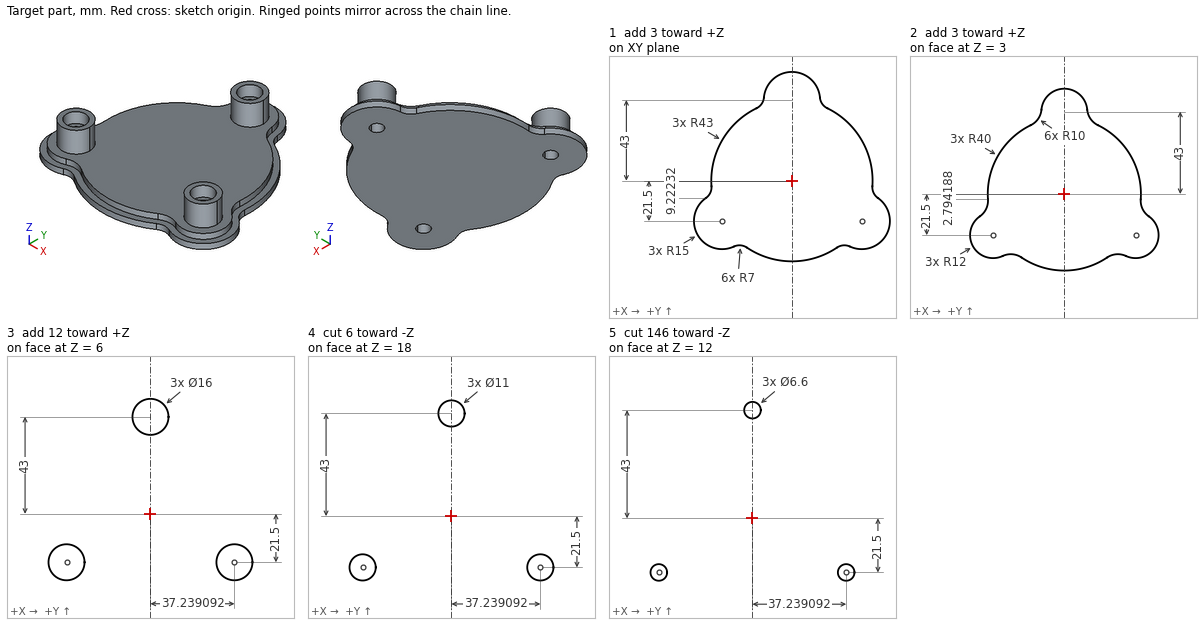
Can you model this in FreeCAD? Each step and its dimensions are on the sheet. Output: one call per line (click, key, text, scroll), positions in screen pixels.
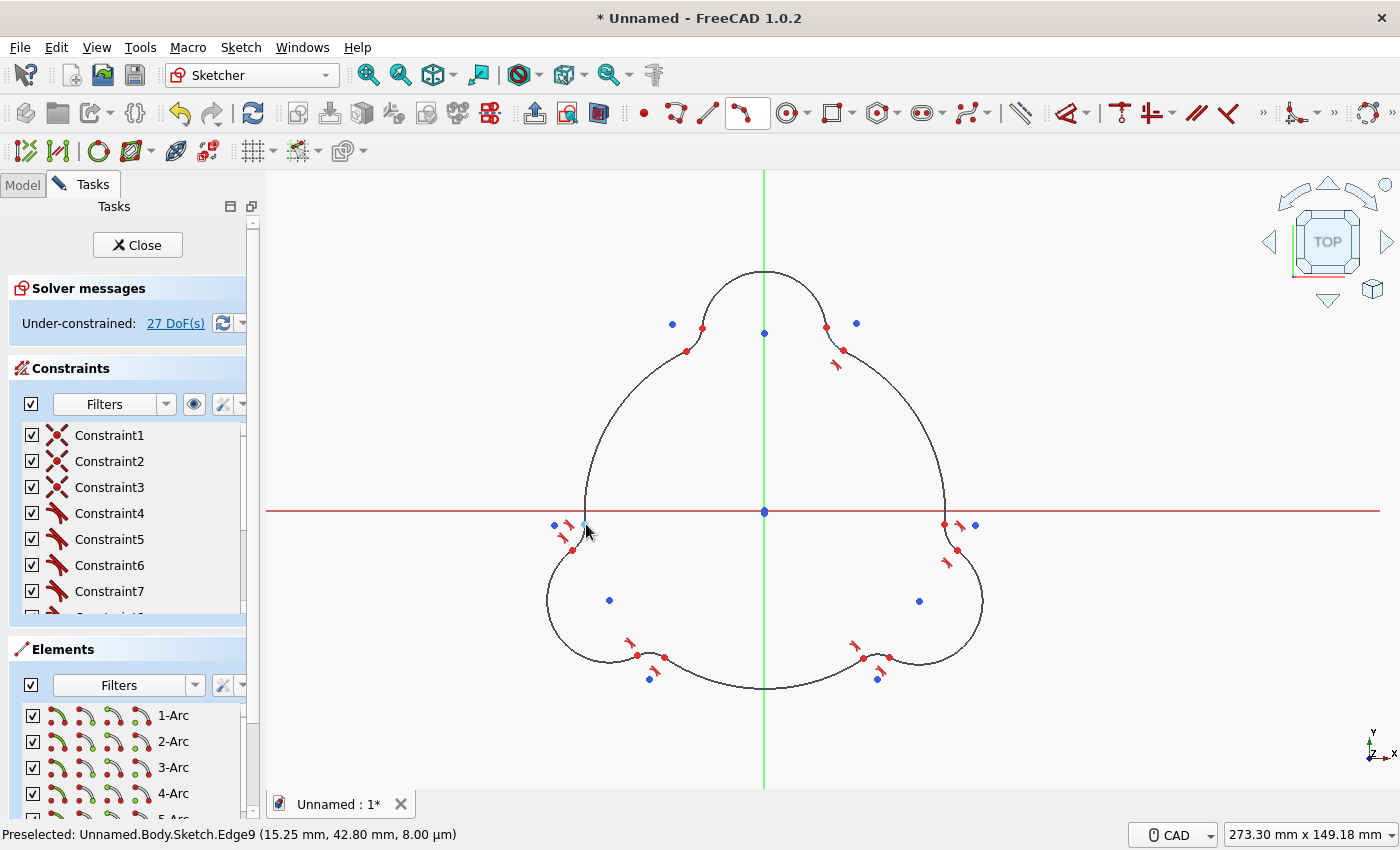
click(799, 282)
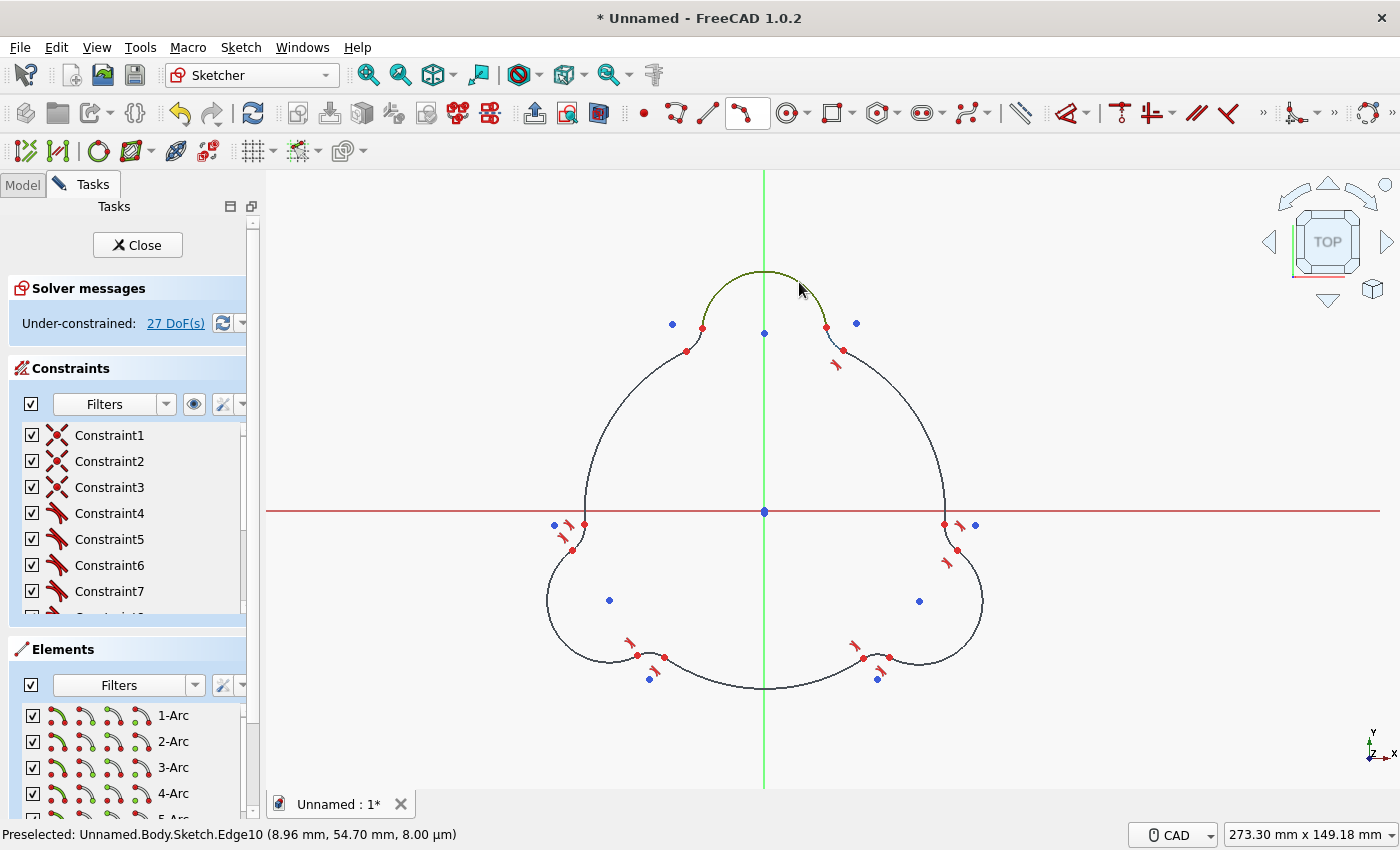
key(t)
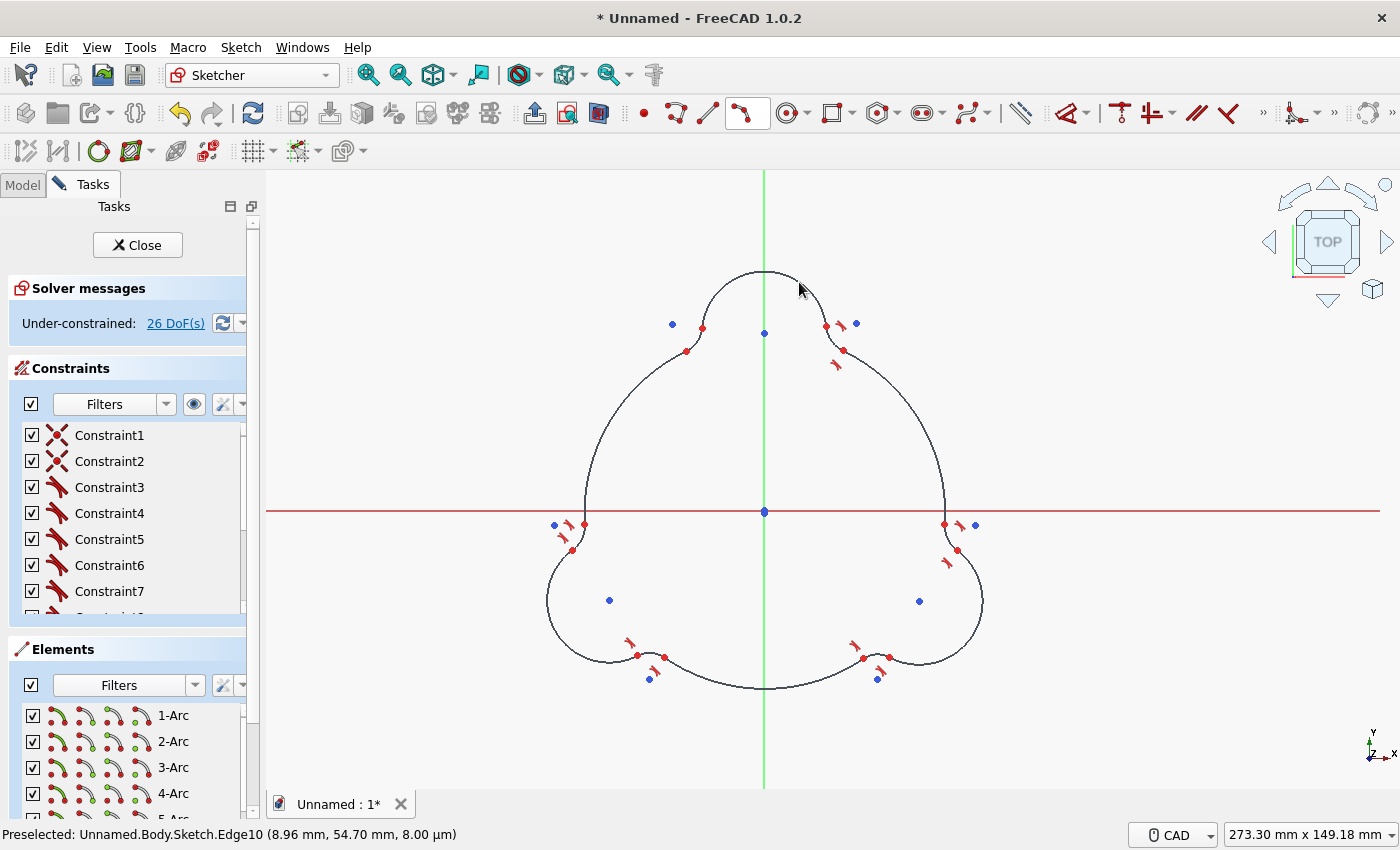
click(798, 282)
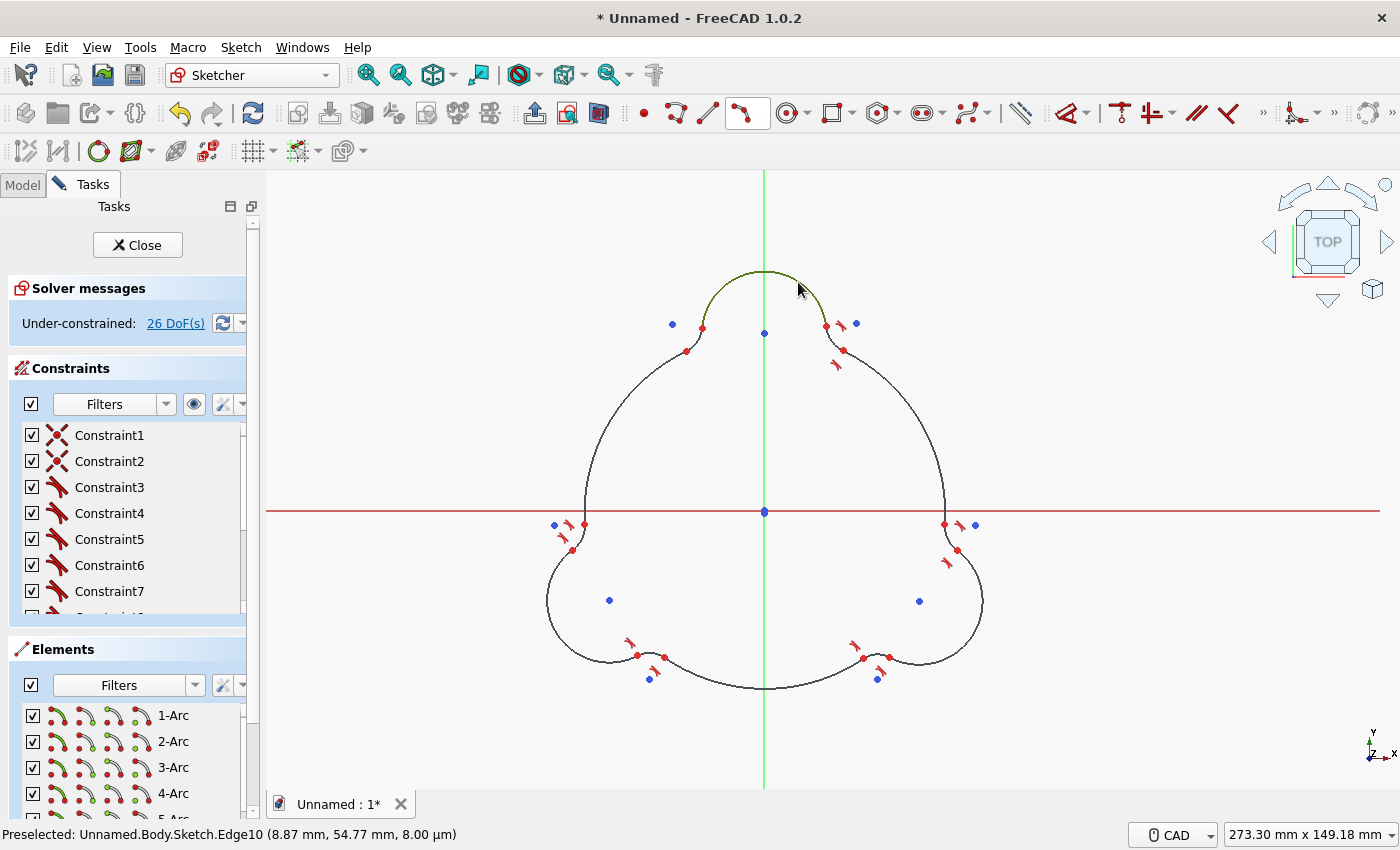
click(697, 342)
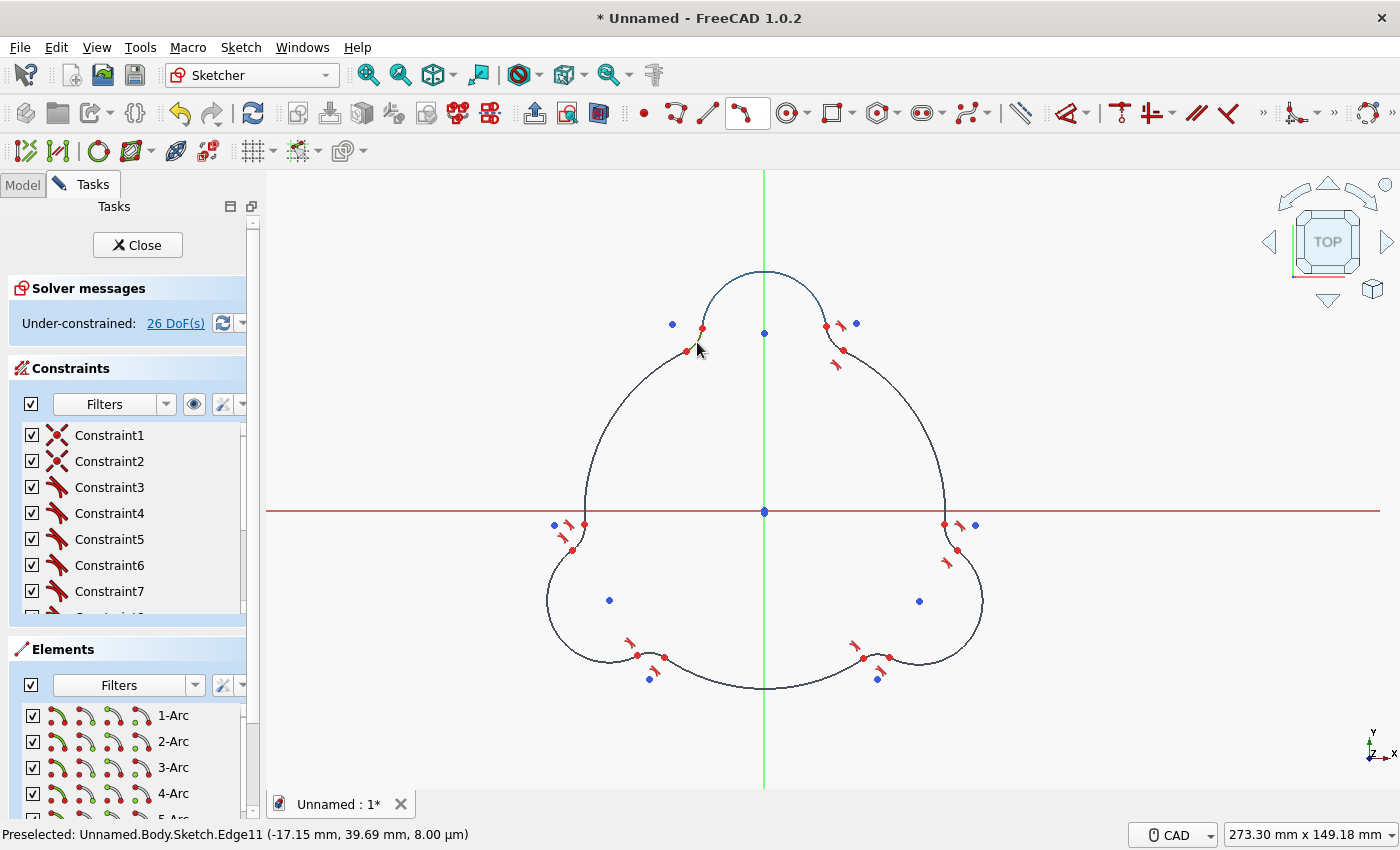
key(t)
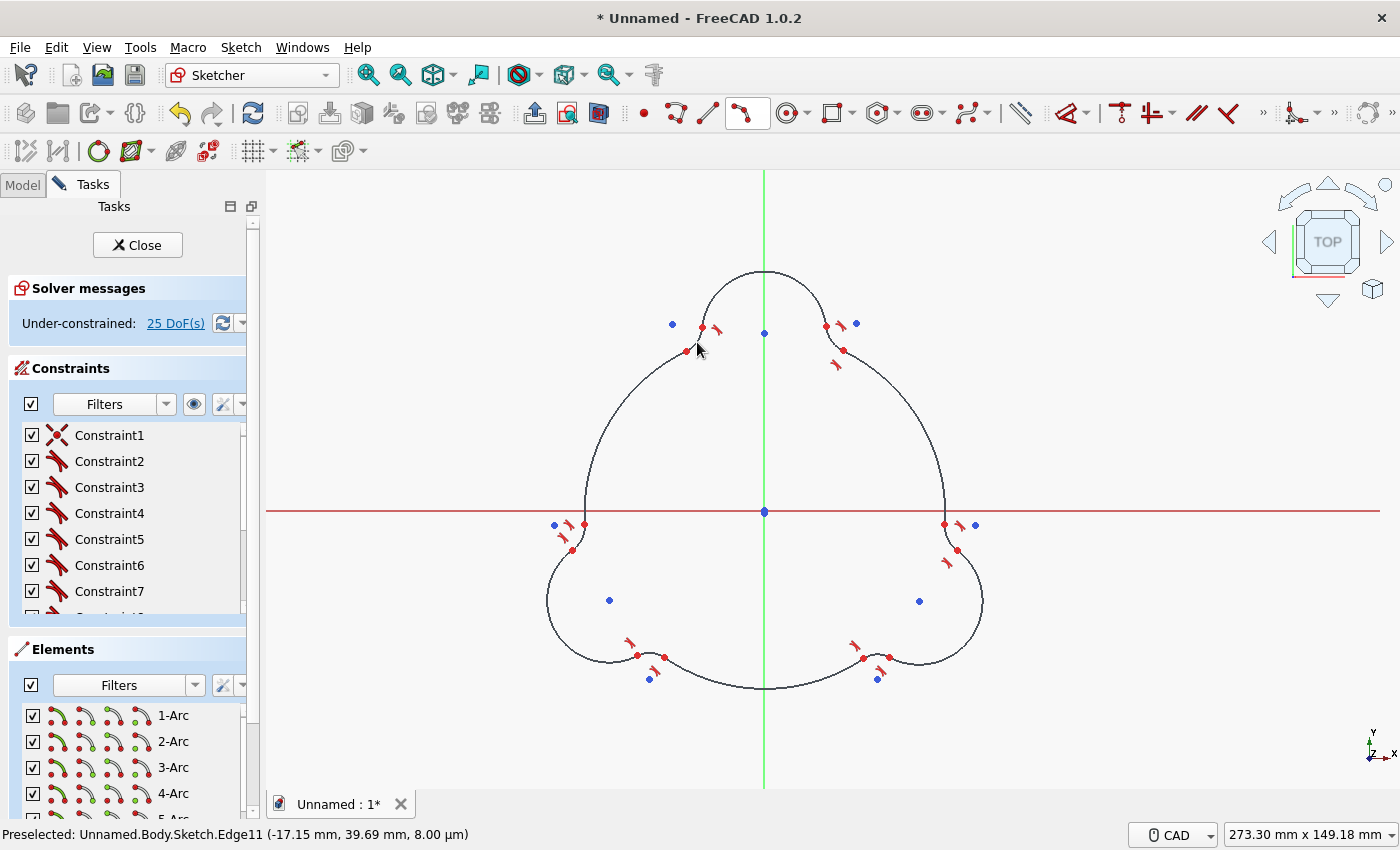
click(697, 342)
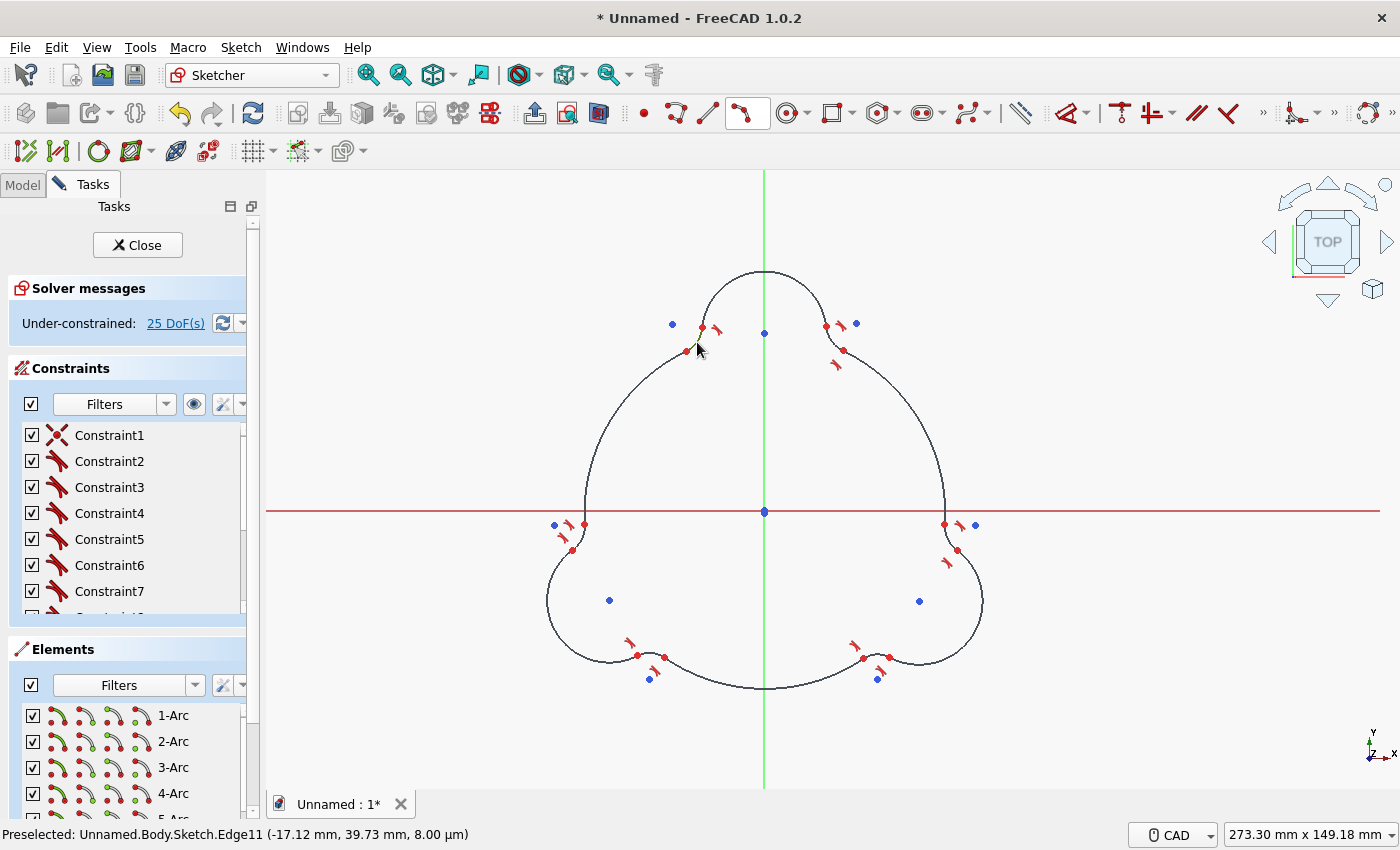
click(635, 389)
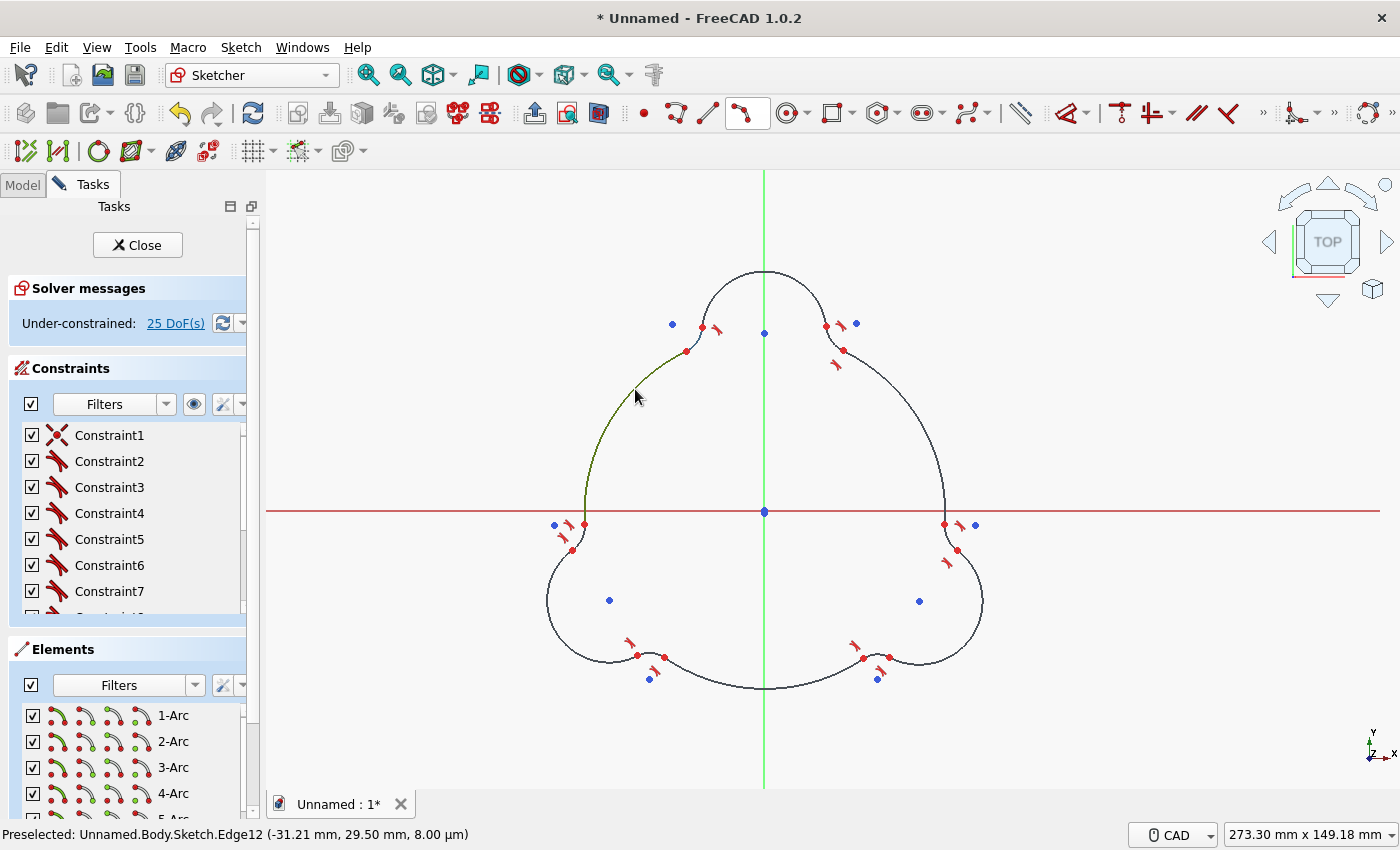
key(t)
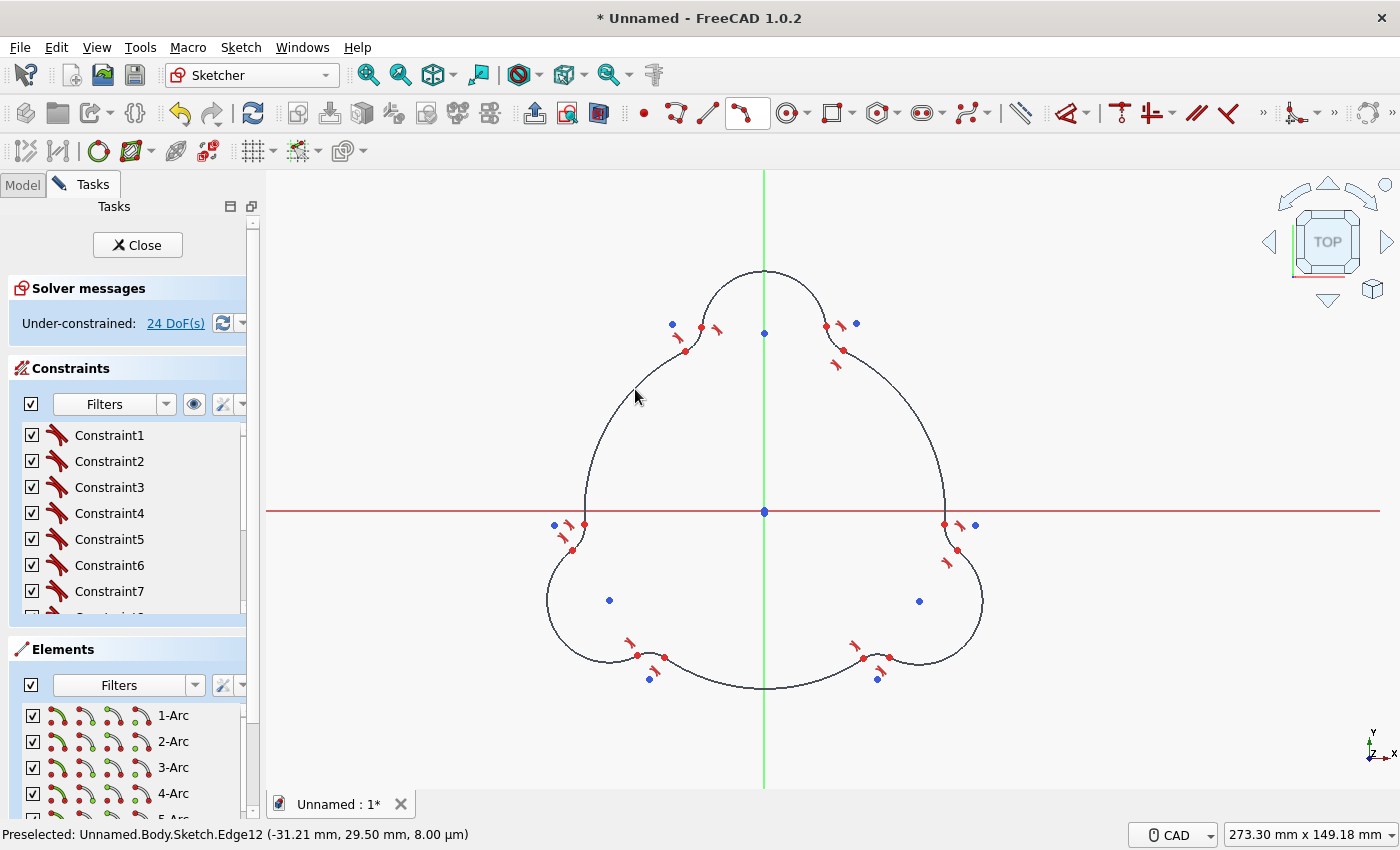
click(722, 684)